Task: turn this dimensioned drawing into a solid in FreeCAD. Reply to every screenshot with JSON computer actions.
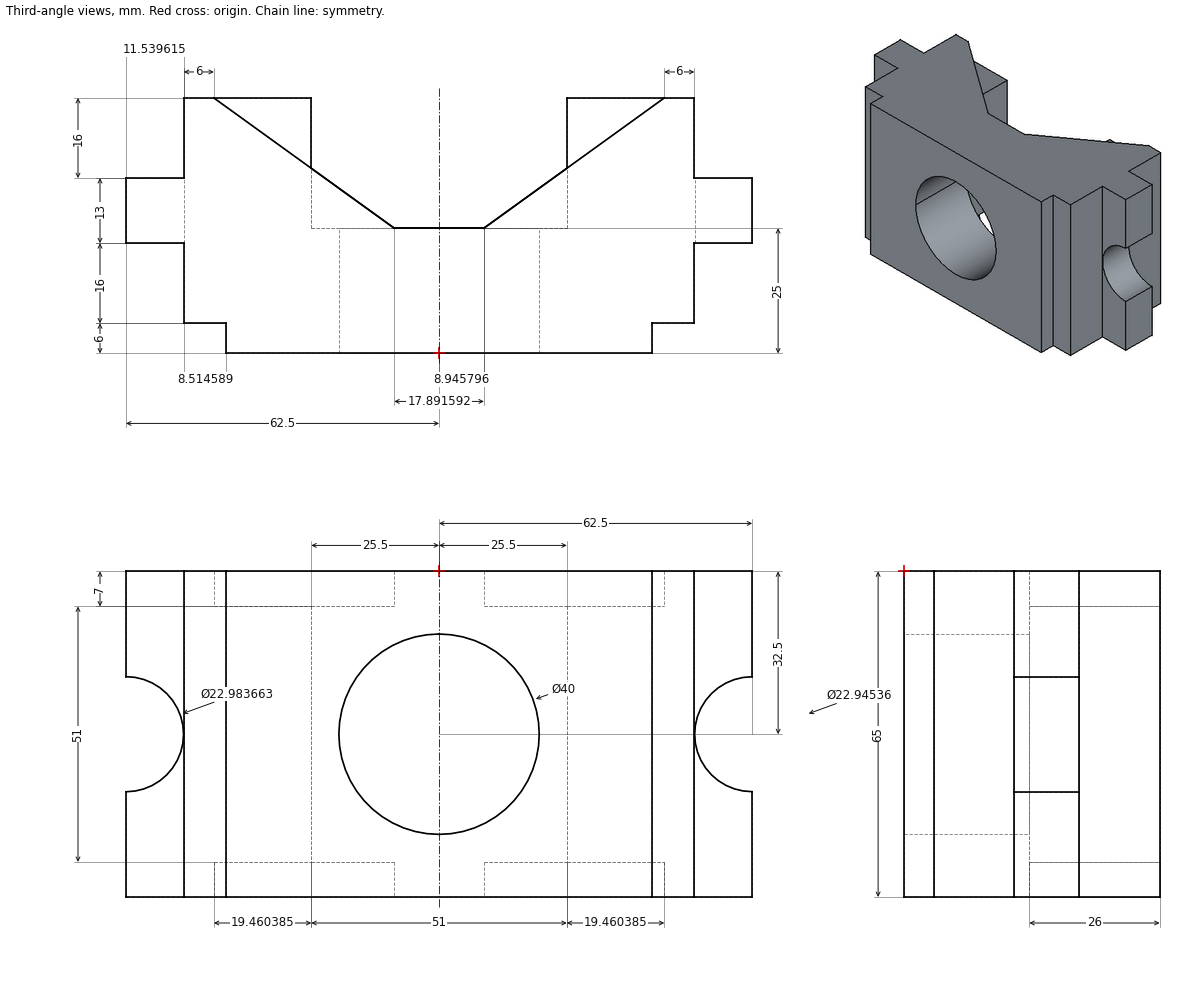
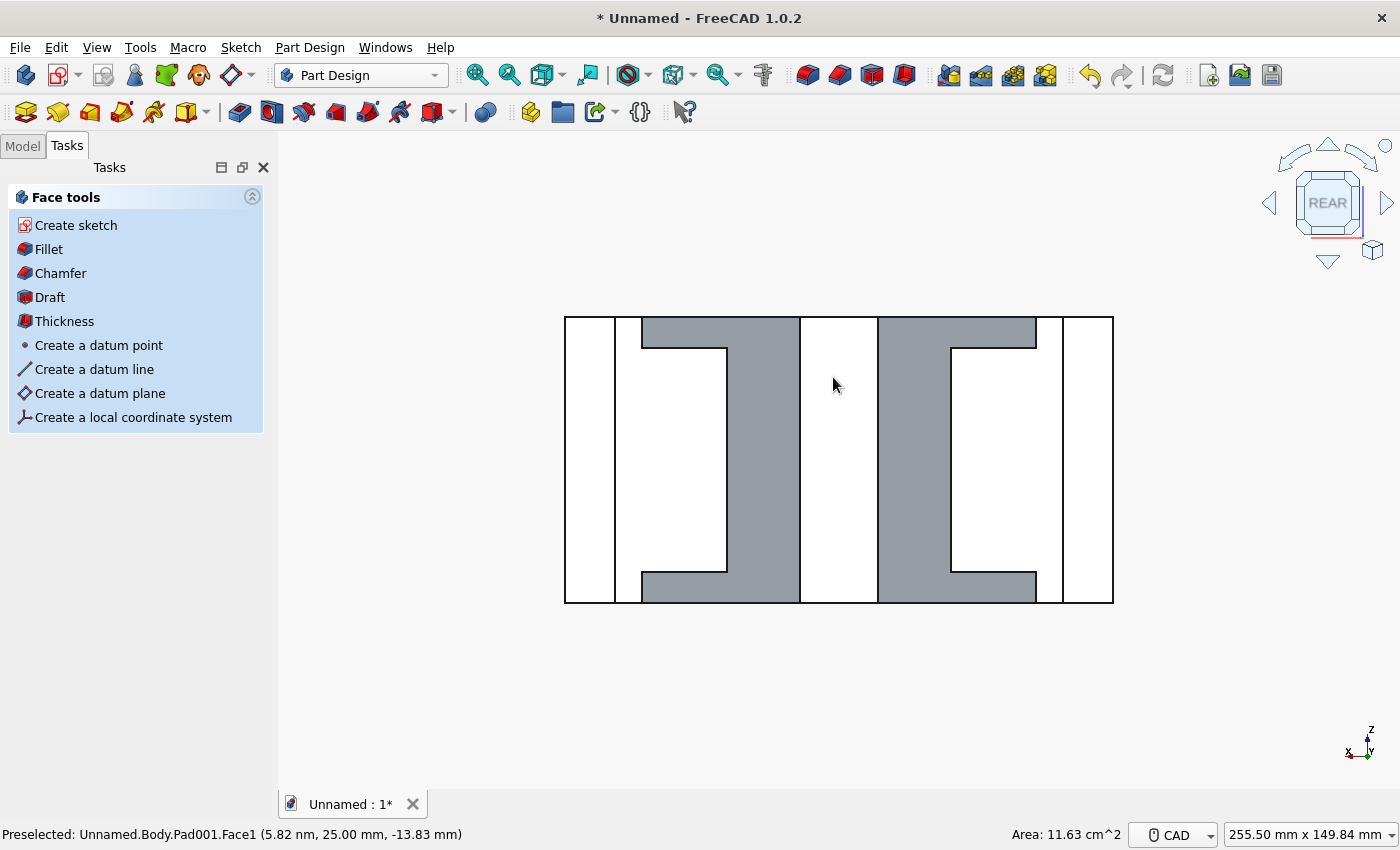
{"action": "left_click", "coordinate": [58, 76]}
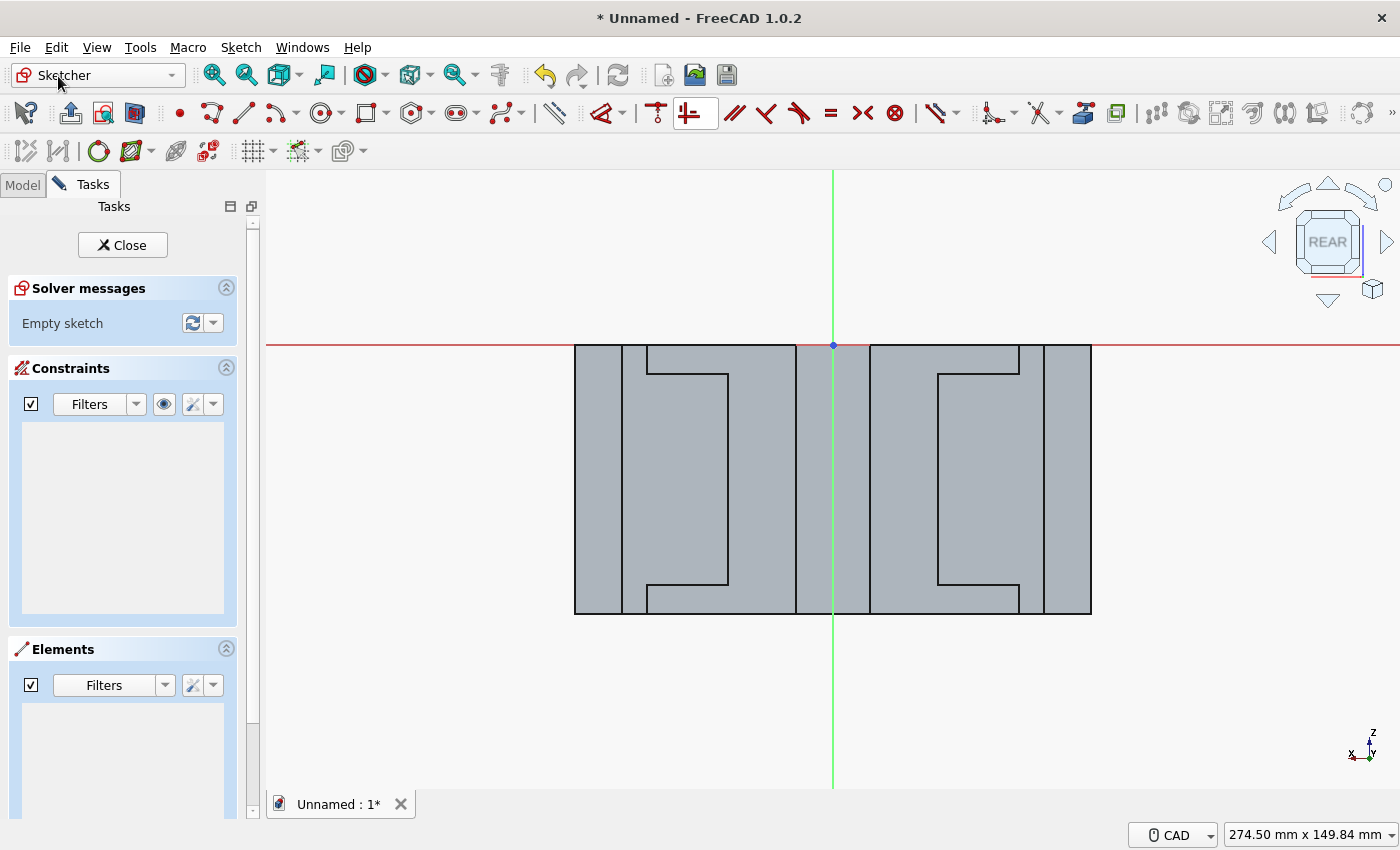
{"action": "left_click", "coordinate": [136, 114]}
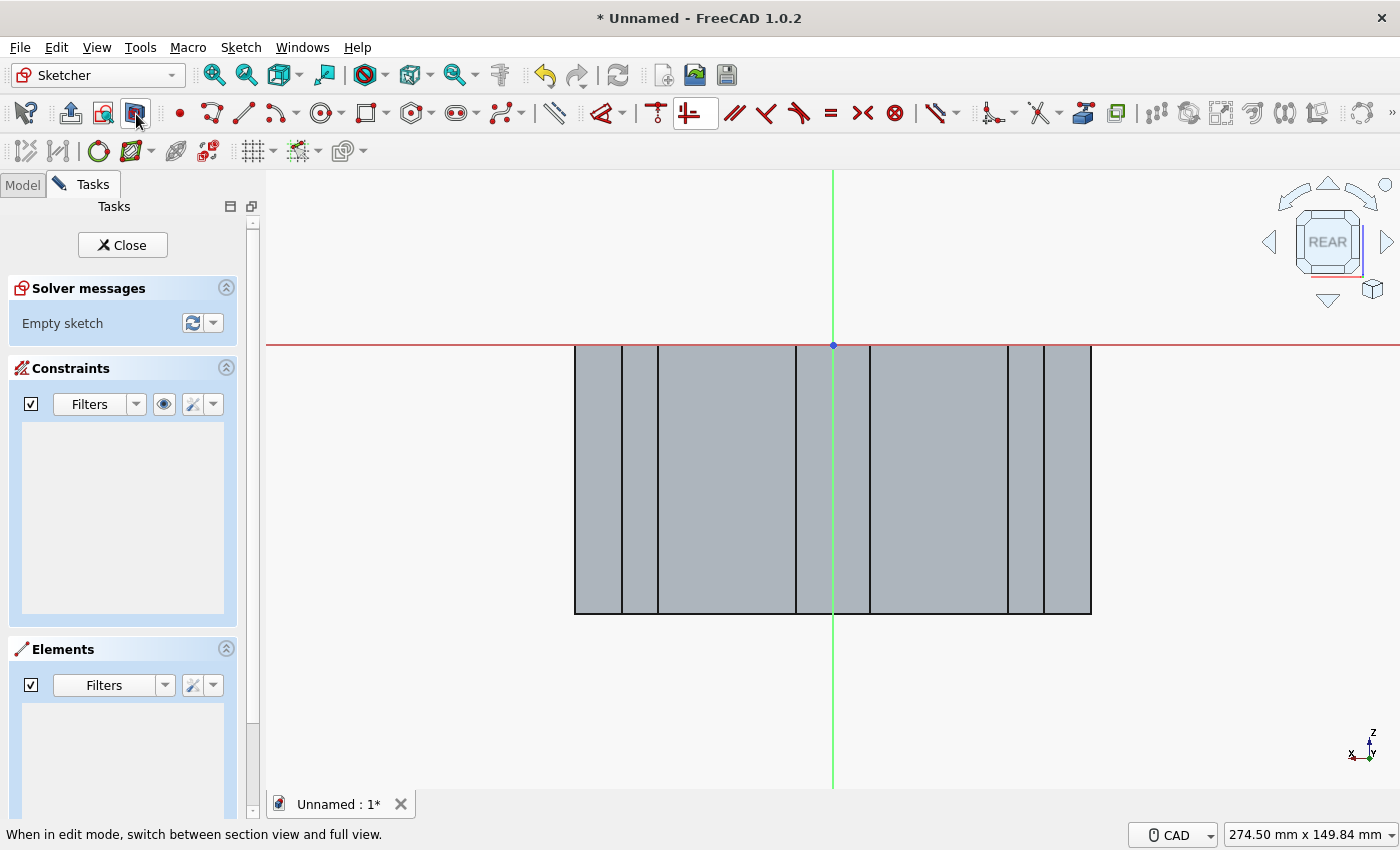
{"action": "scroll", "coordinate": [916, 447], "scroll_direction": "up", "scroll_amount": 3}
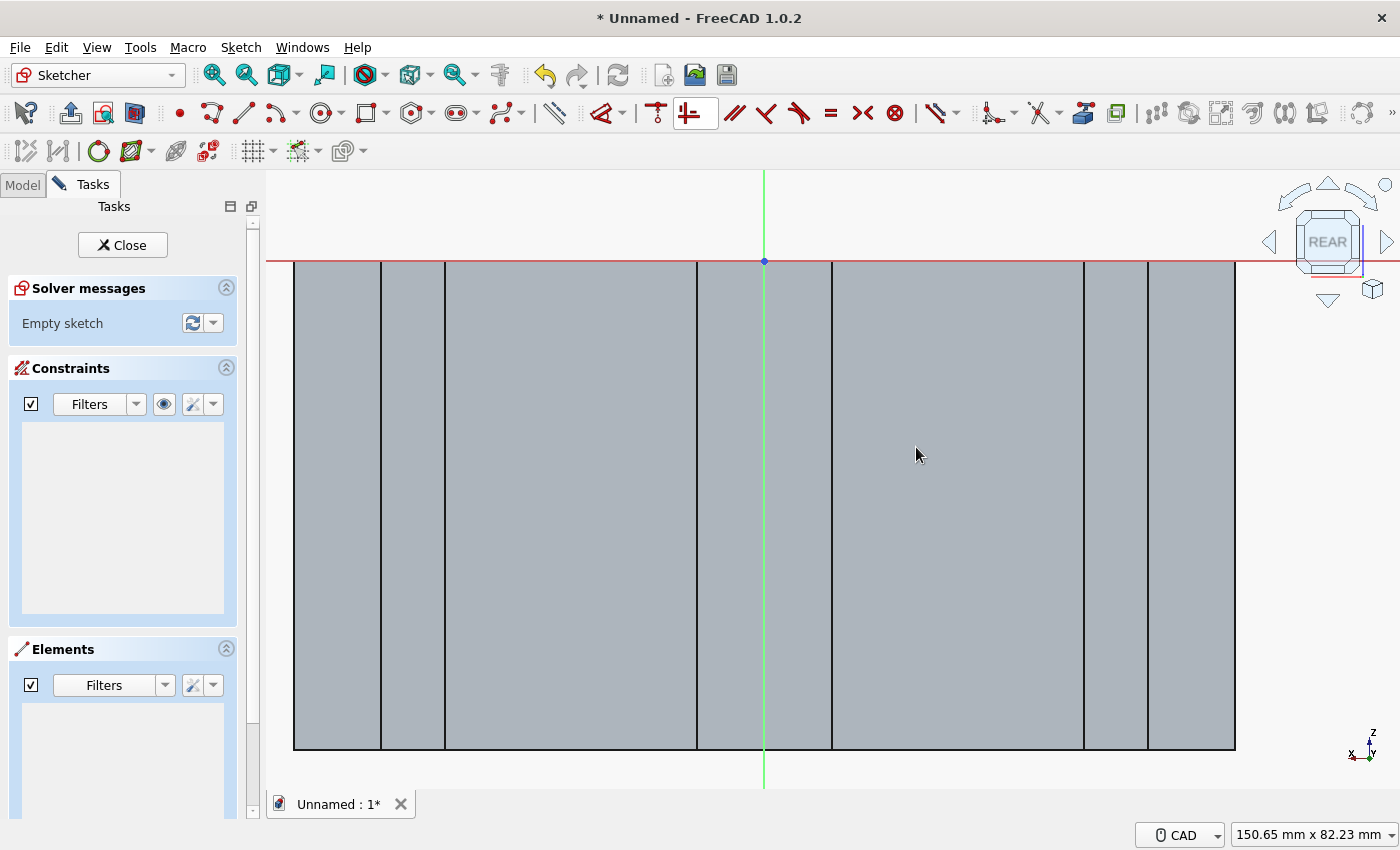
{"action": "left_click", "coordinate": [366, 114]}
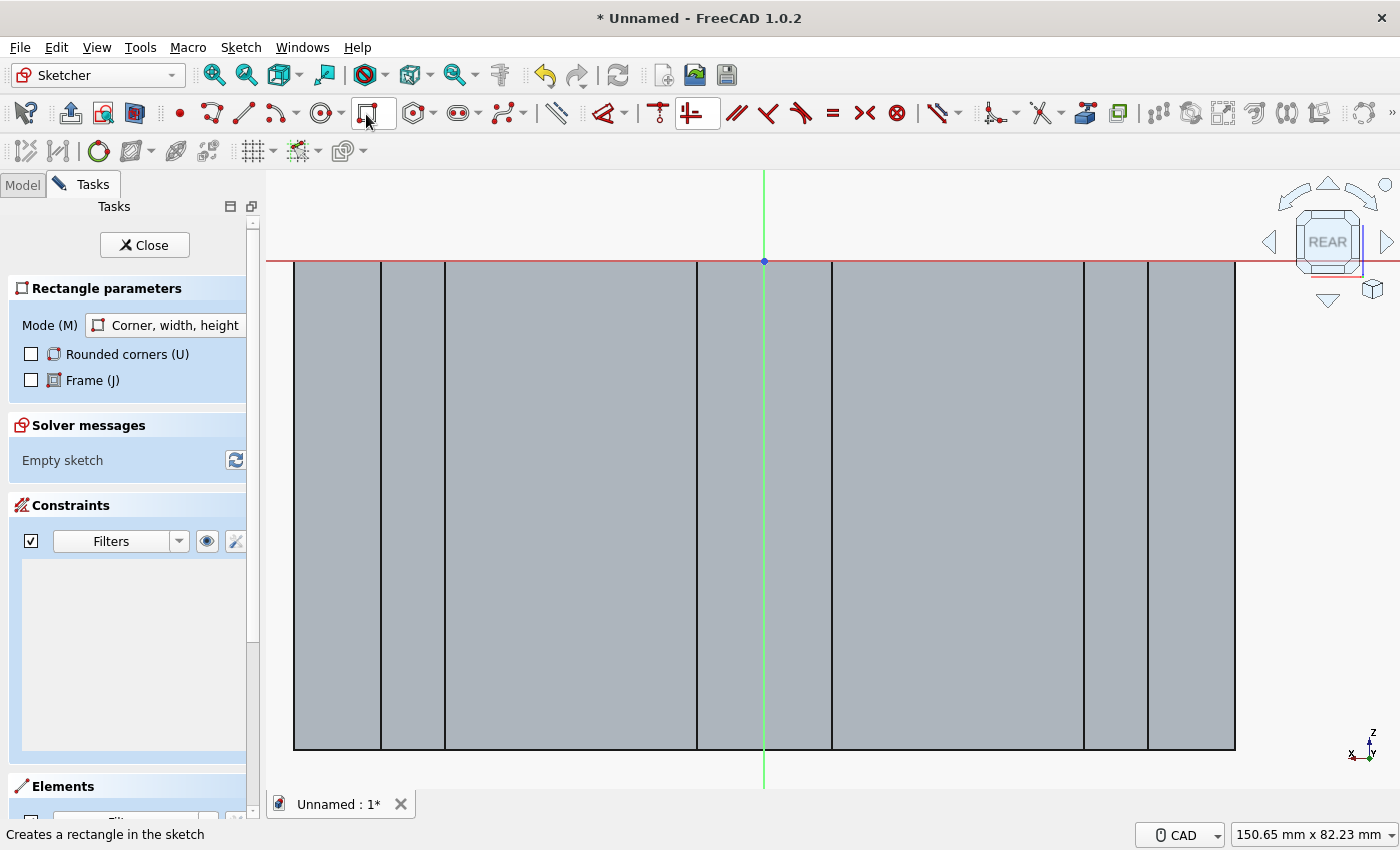
{"action": "left_click", "coordinate": [572, 314]}
{"action": "mouse_move", "coordinate": [956, 698]}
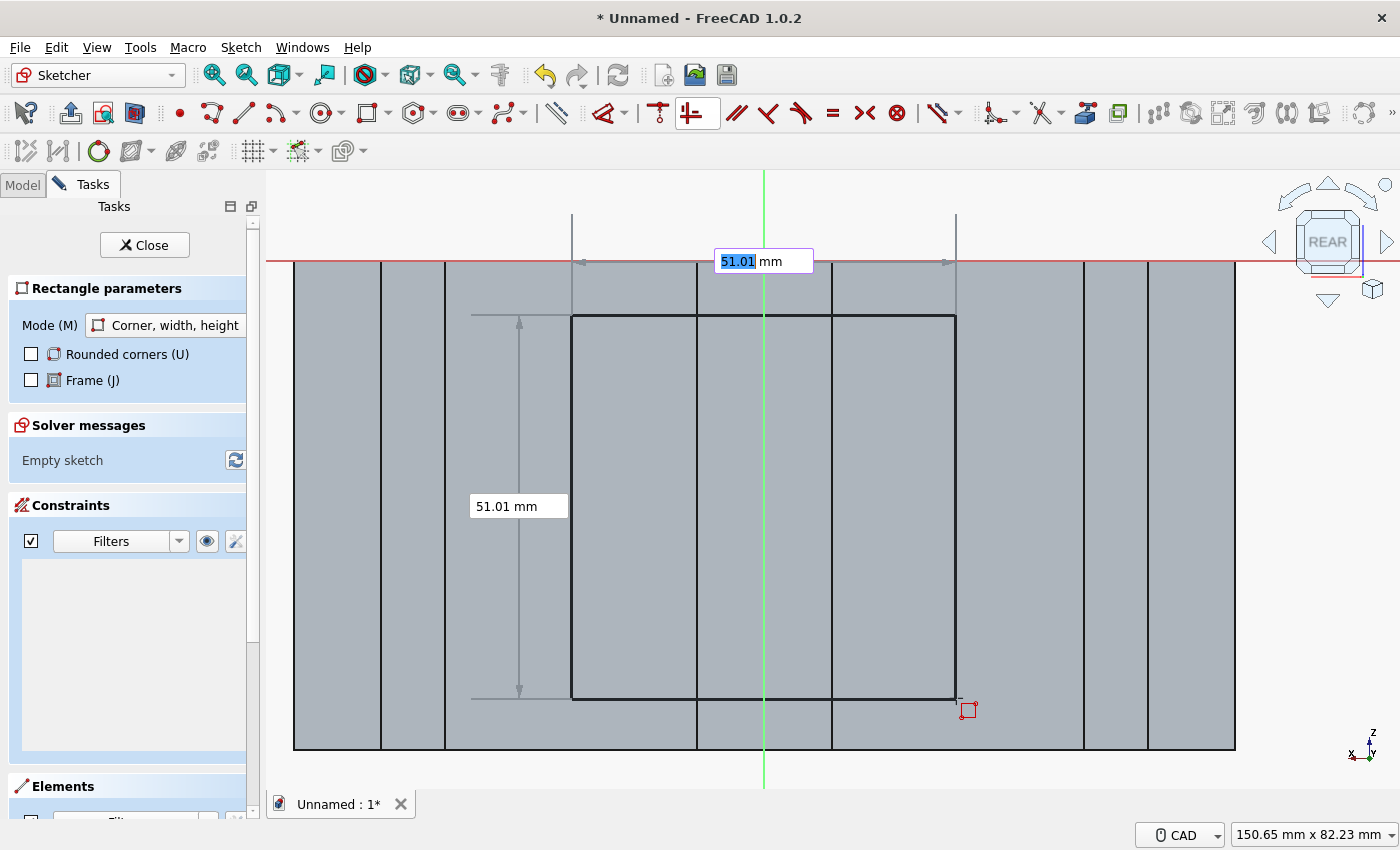
{"action": "type", "text": "51"}
{"action": "key", "text": "Tab"}
{"action": "type", "text": "51"}
{"action": "key", "text": "Return"}
{"action": "key", "text": "Escape"}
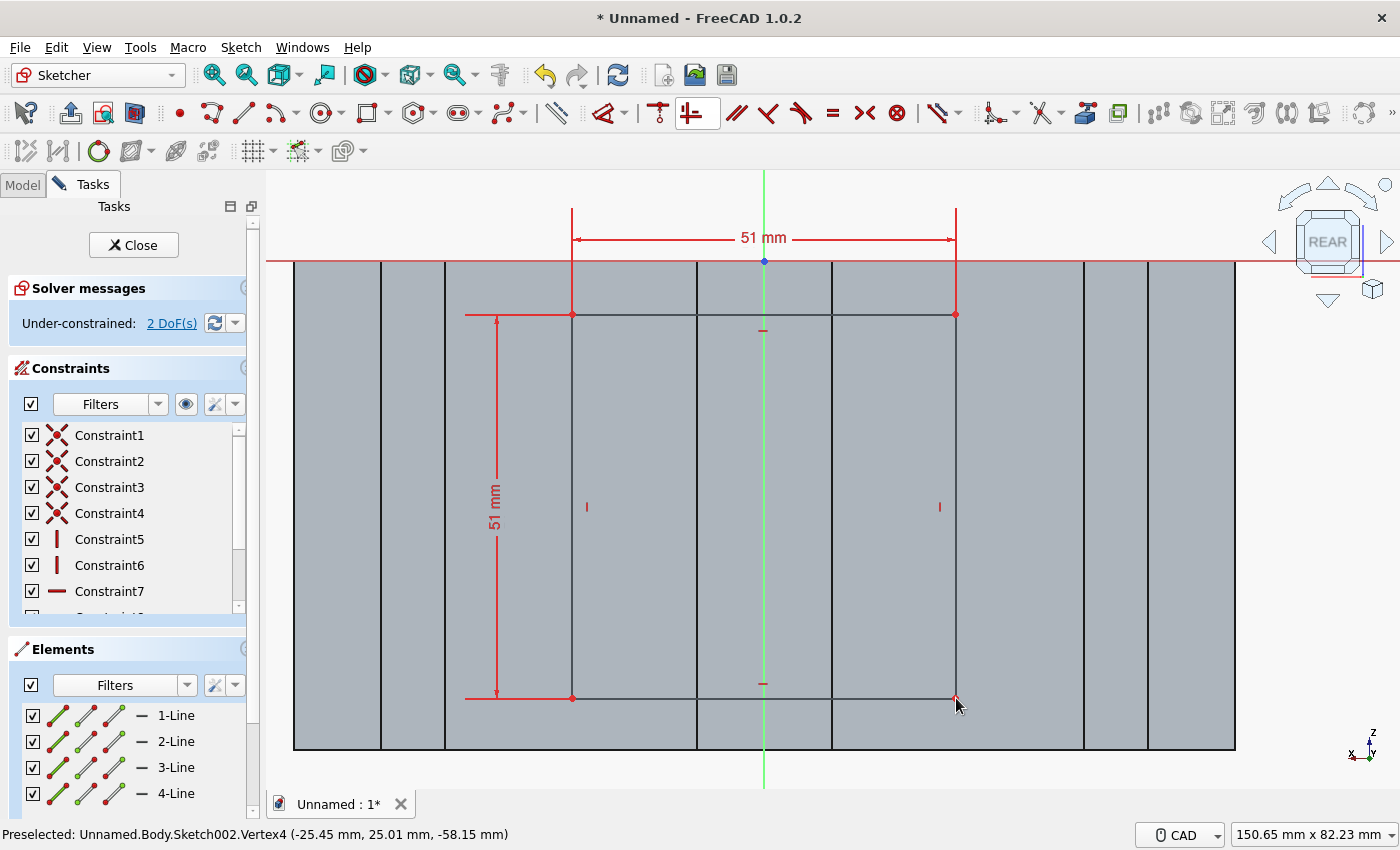
{"action": "left_click", "coordinate": [604, 114]}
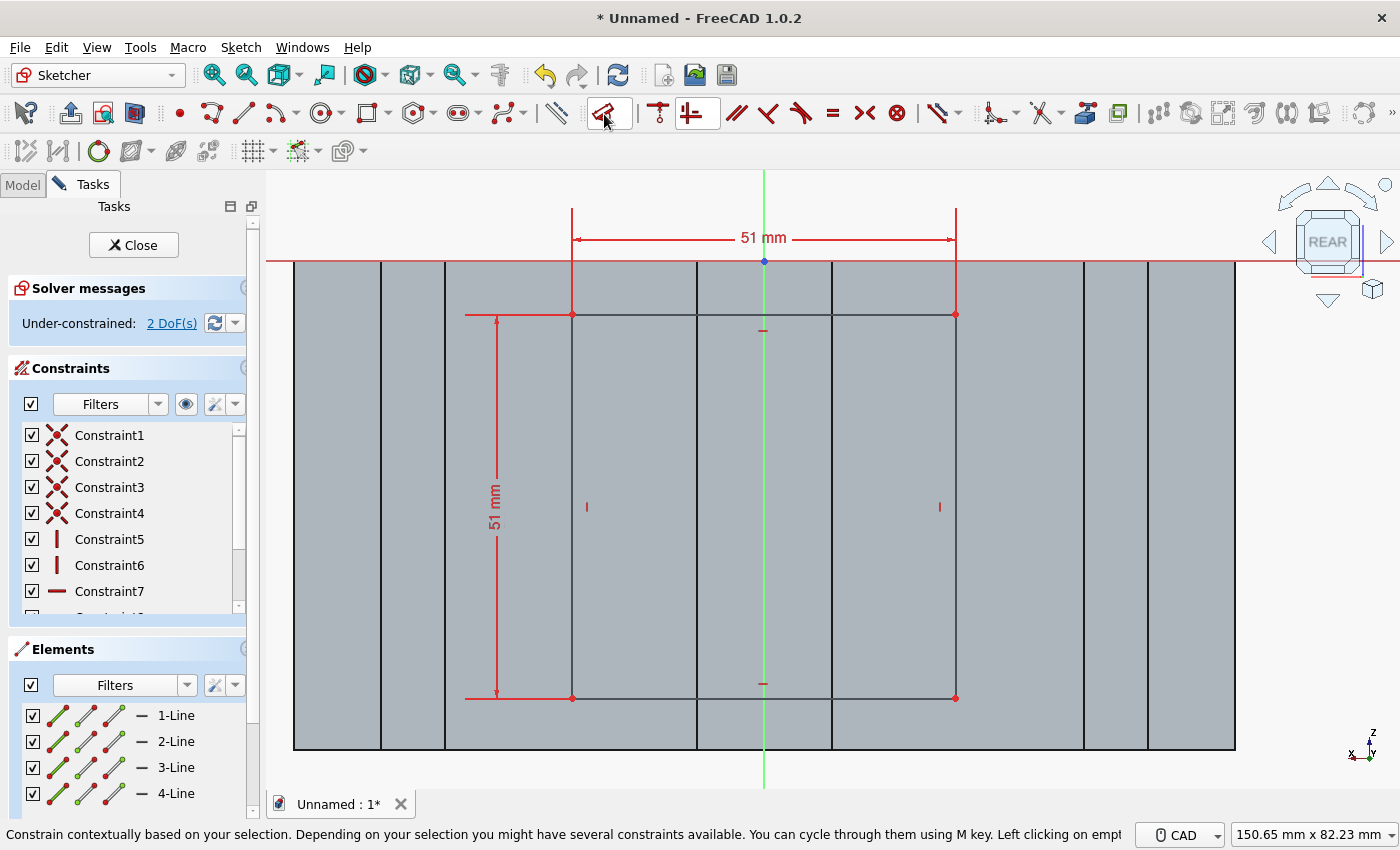
{"action": "left_click", "coordinate": [572, 315]}
{"action": "left_click", "coordinate": [538, 288]}